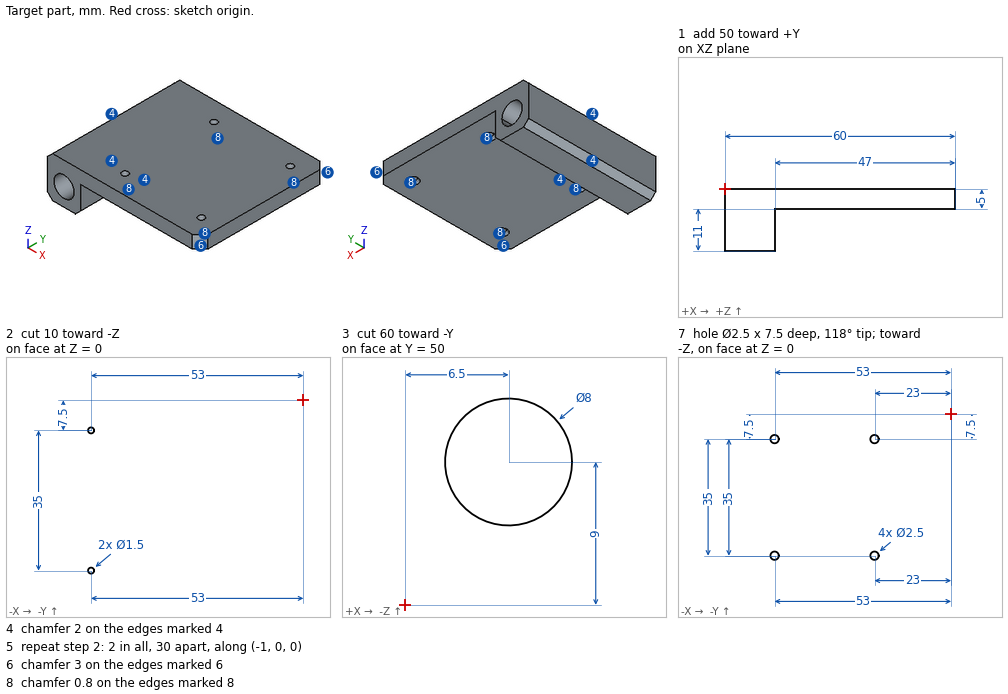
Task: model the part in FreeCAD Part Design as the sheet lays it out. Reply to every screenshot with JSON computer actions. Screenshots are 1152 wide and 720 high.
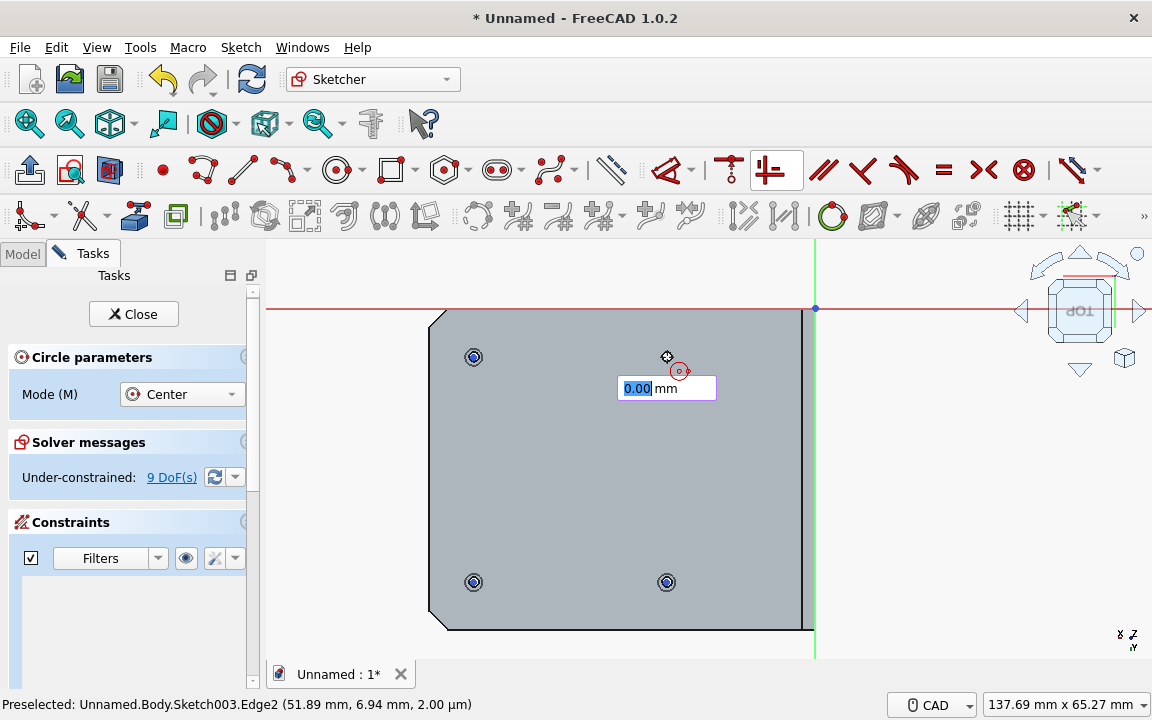
{"action": "scroll", "coordinate": [673, 351], "scroll_direction": "up", "scroll_amount": 4}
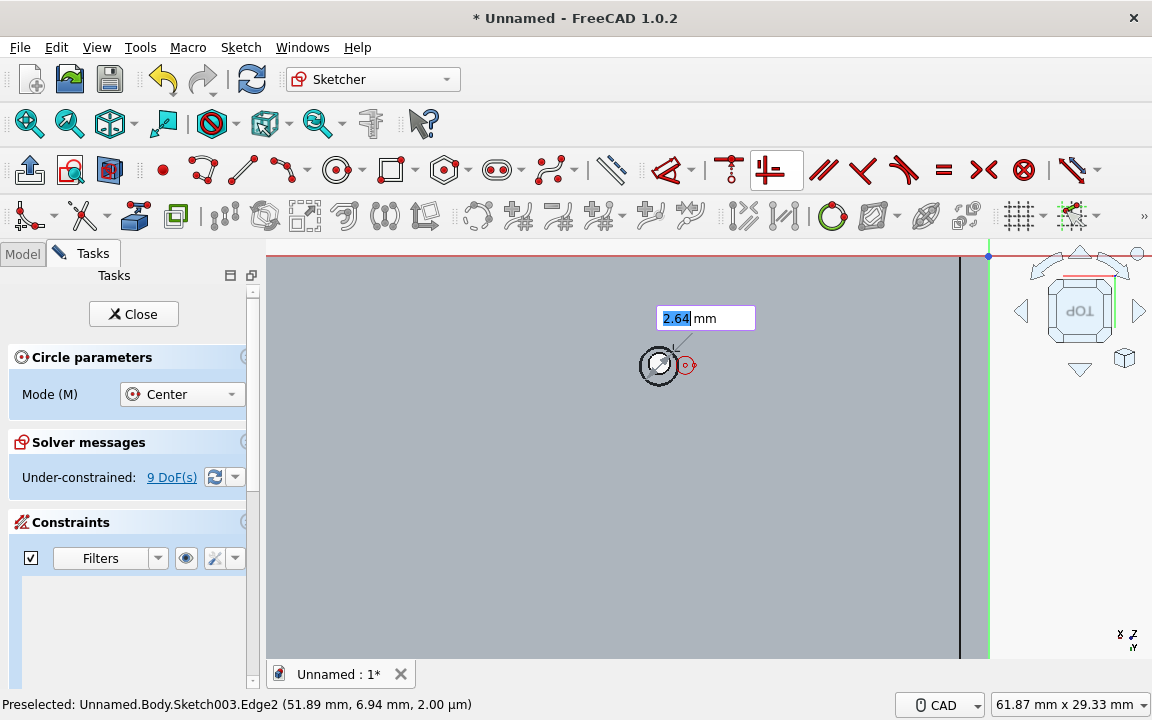
{"action": "left_click", "coordinate": [672, 351]}
{"action": "key", "text": "Escape"}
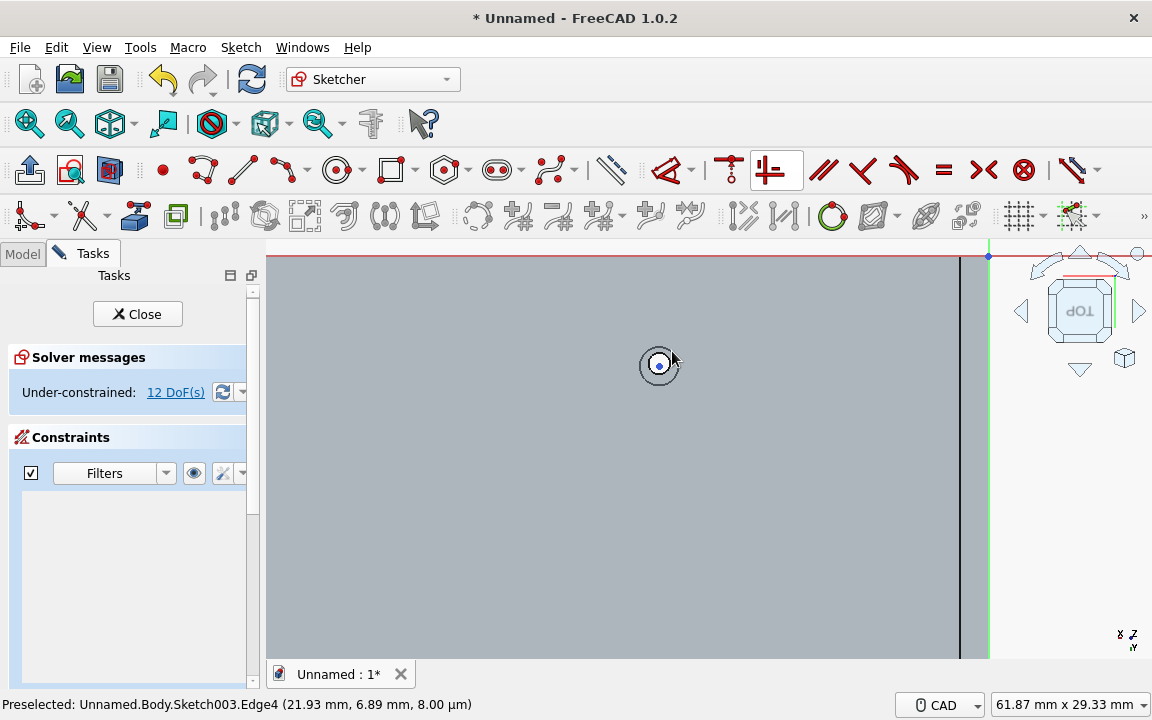
{"action": "scroll", "coordinate": [673, 351], "scroll_direction": "down", "scroll_amount": 4}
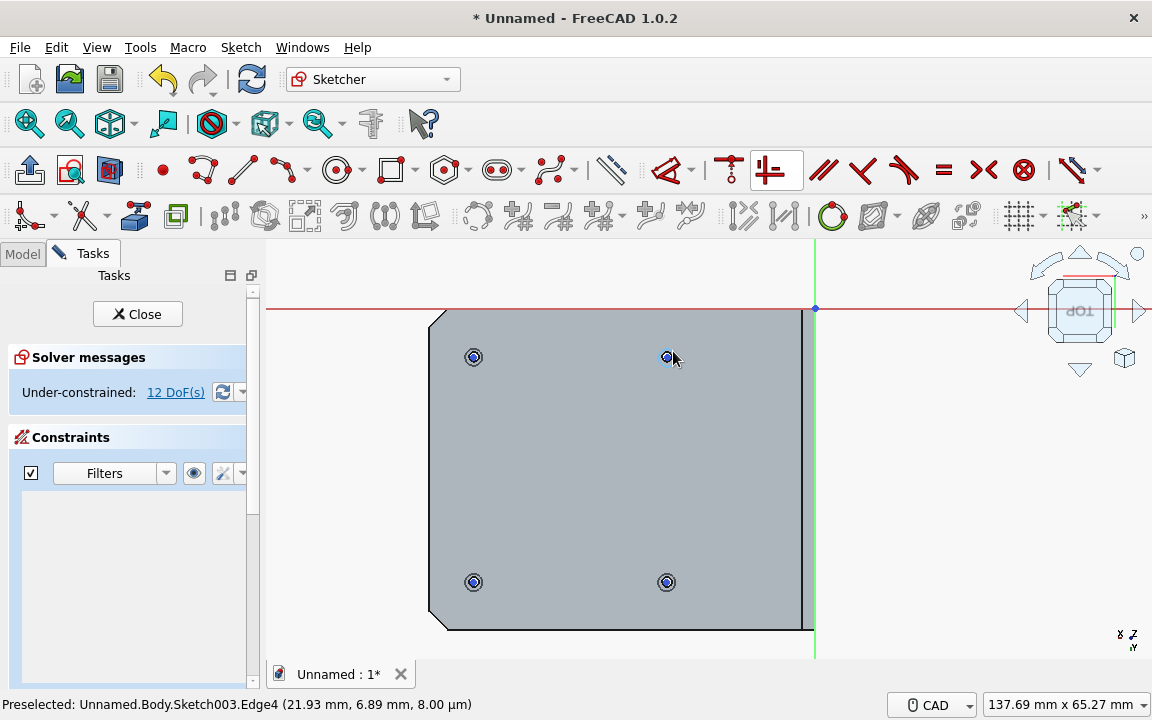
{"action": "scroll", "coordinate": [673, 576], "scroll_direction": "up", "scroll_amount": 3}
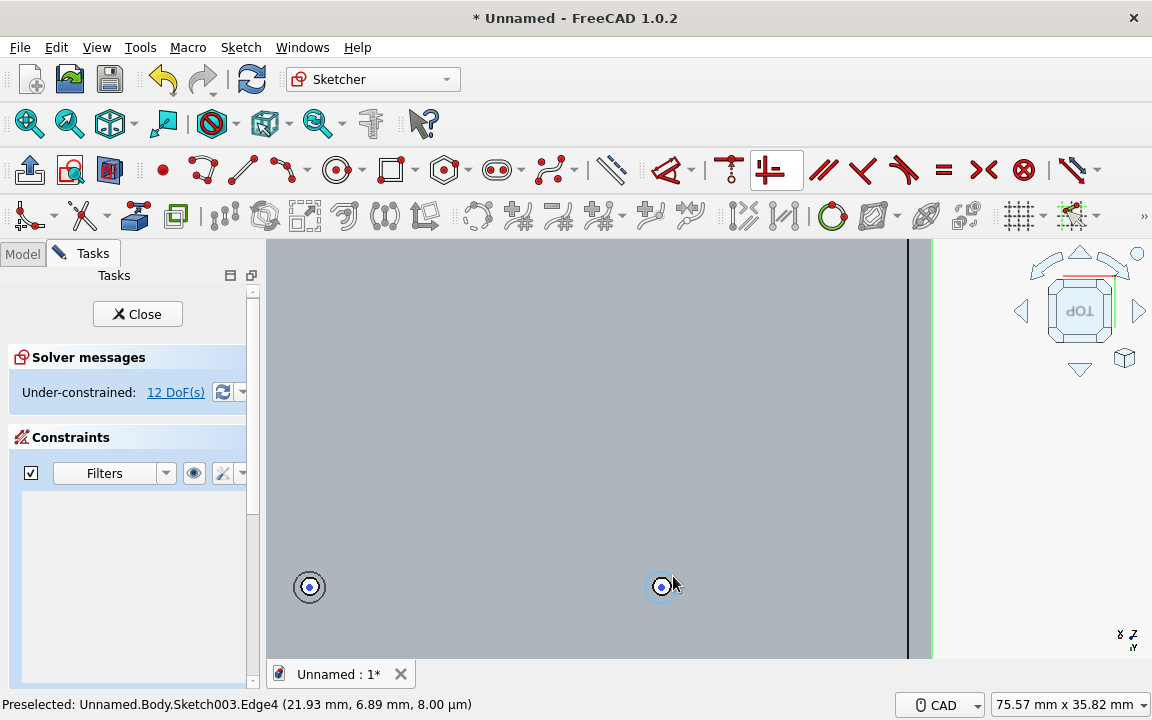
{"action": "left_click", "coordinate": [672, 576]}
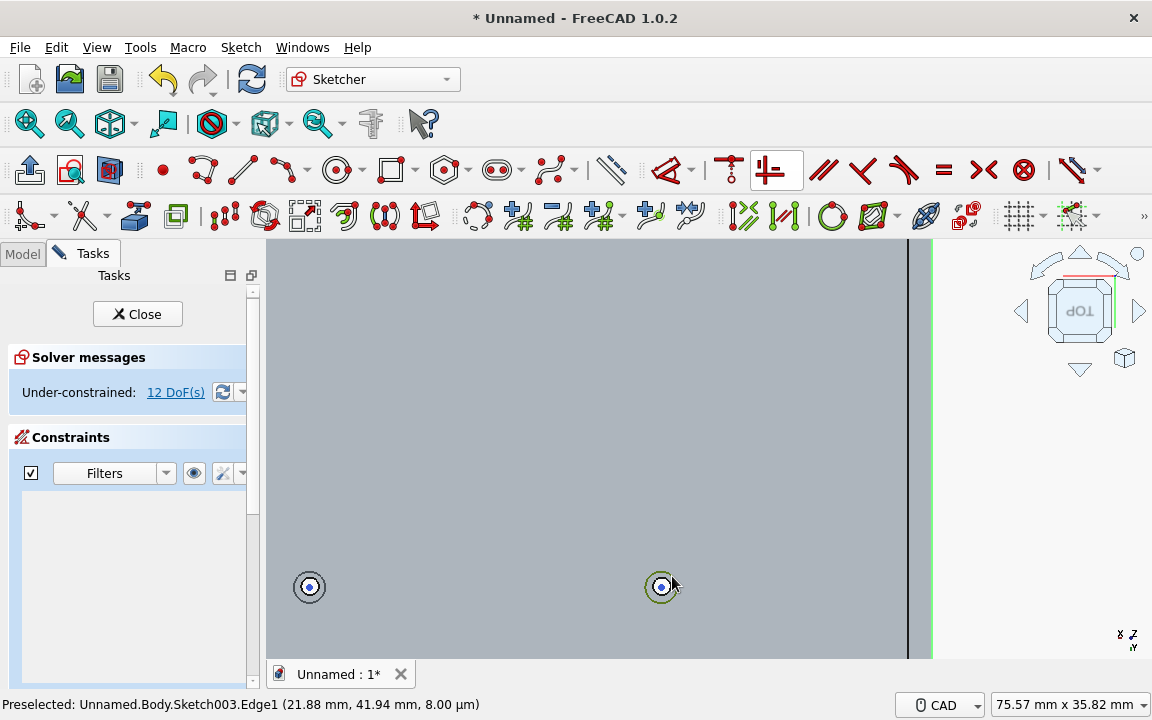
{"action": "left_click", "coordinate": [321, 576]}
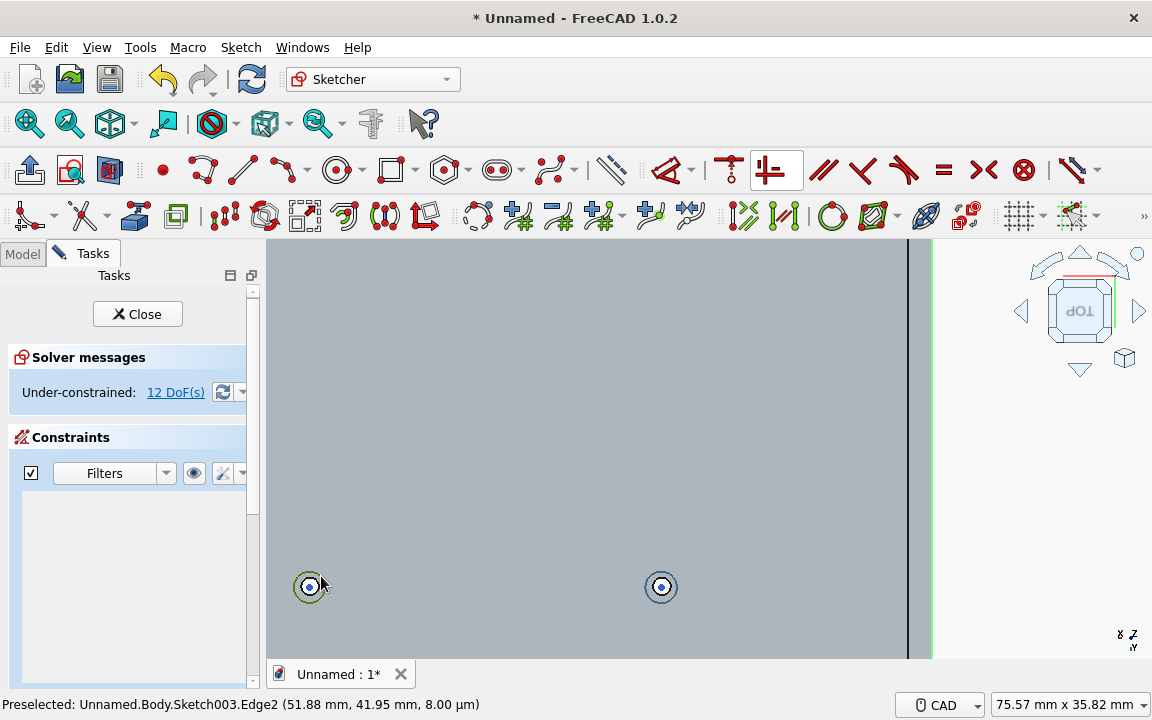
{"action": "scroll", "coordinate": [673, 576], "scroll_direction": "down", "scroll_amount": 3}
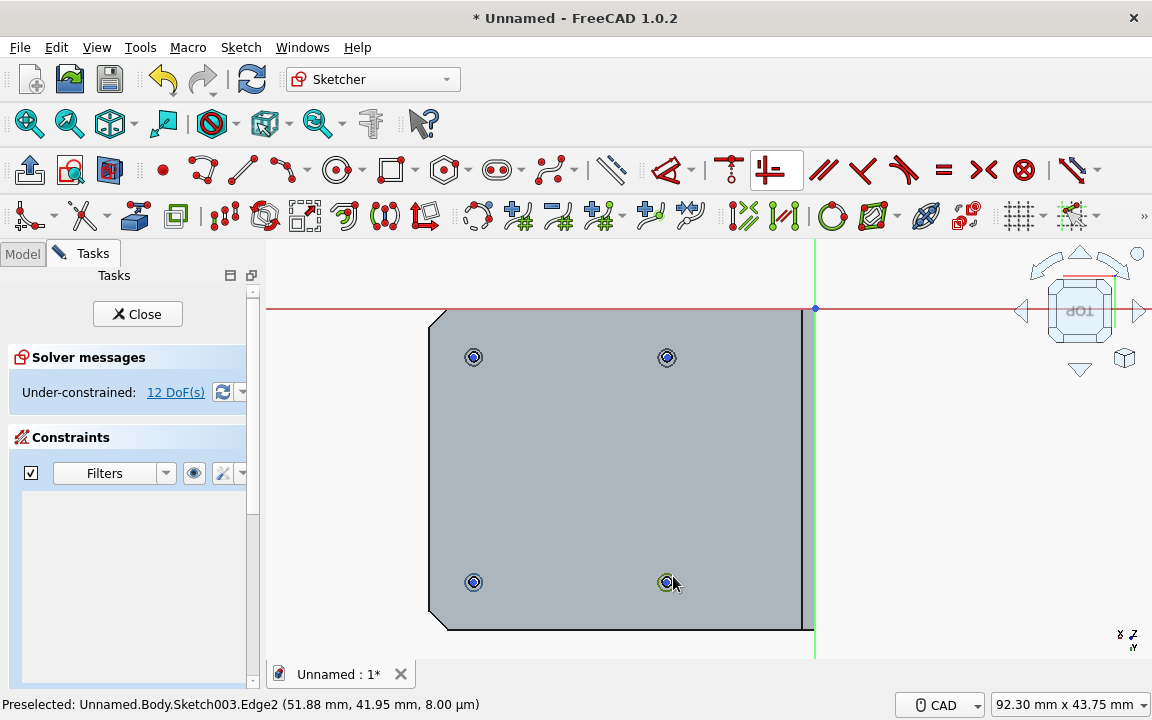
{"action": "scroll", "coordinate": [480, 351], "scroll_direction": "up", "scroll_amount": 3}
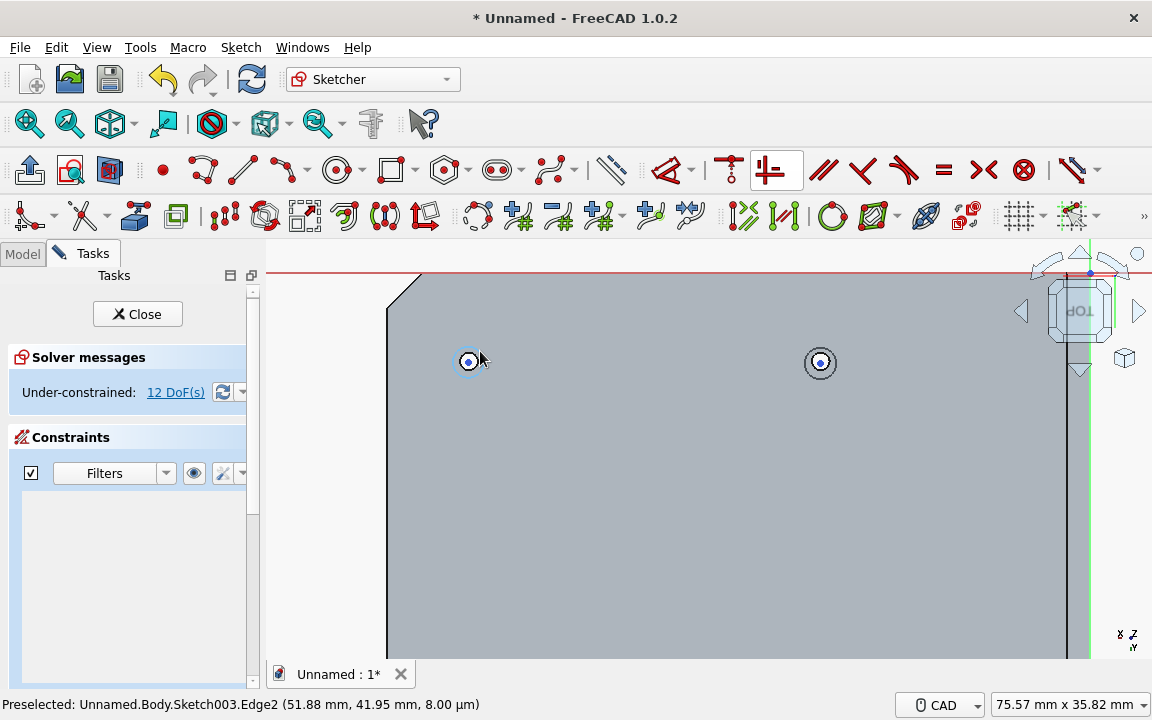
{"action": "left_click", "coordinate": [479, 351]}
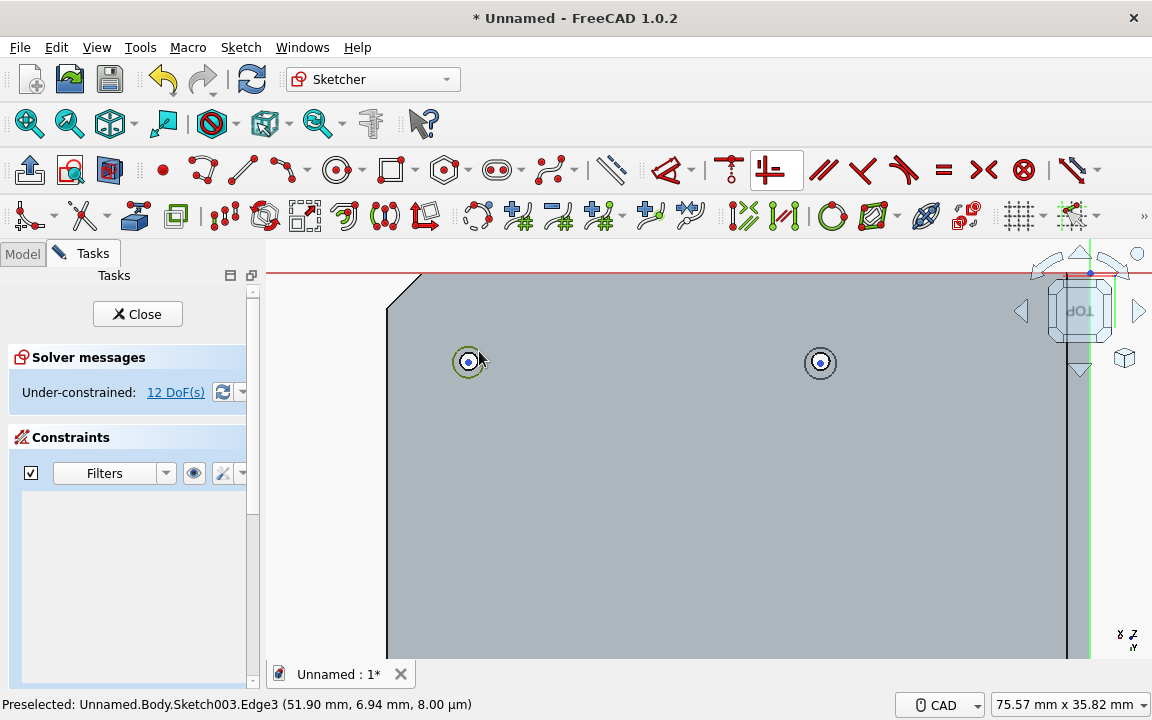
{"action": "left_click", "coordinate": [832, 352]}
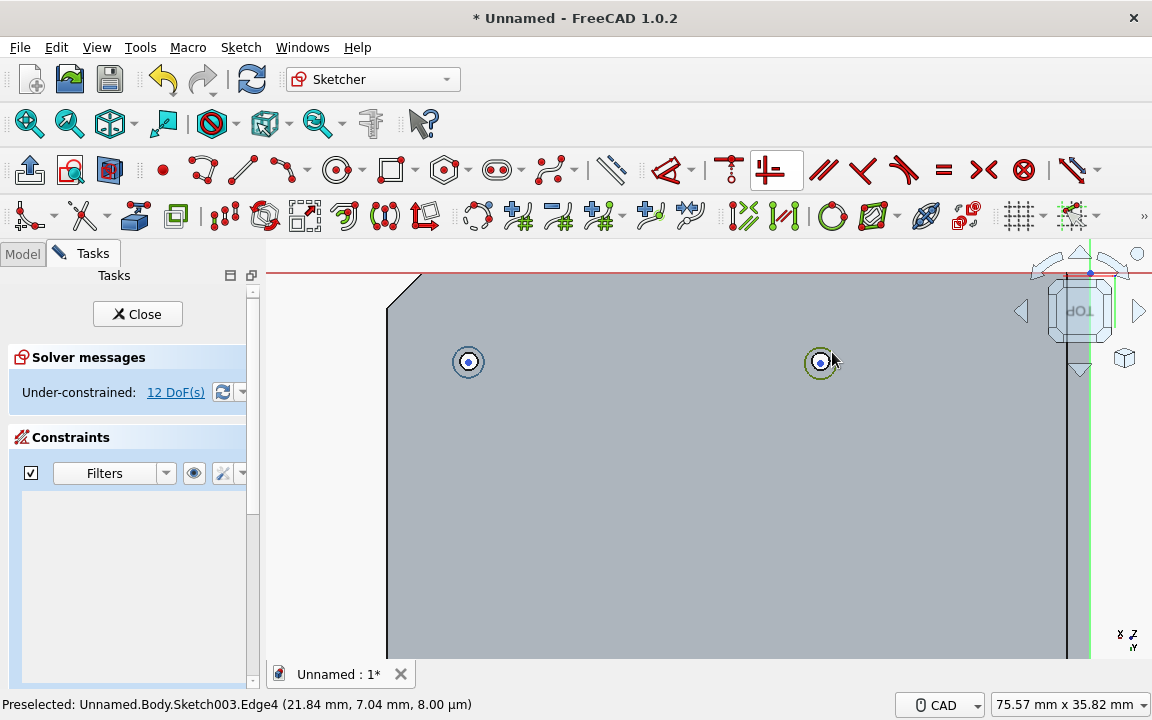
{"action": "key", "text": "e"}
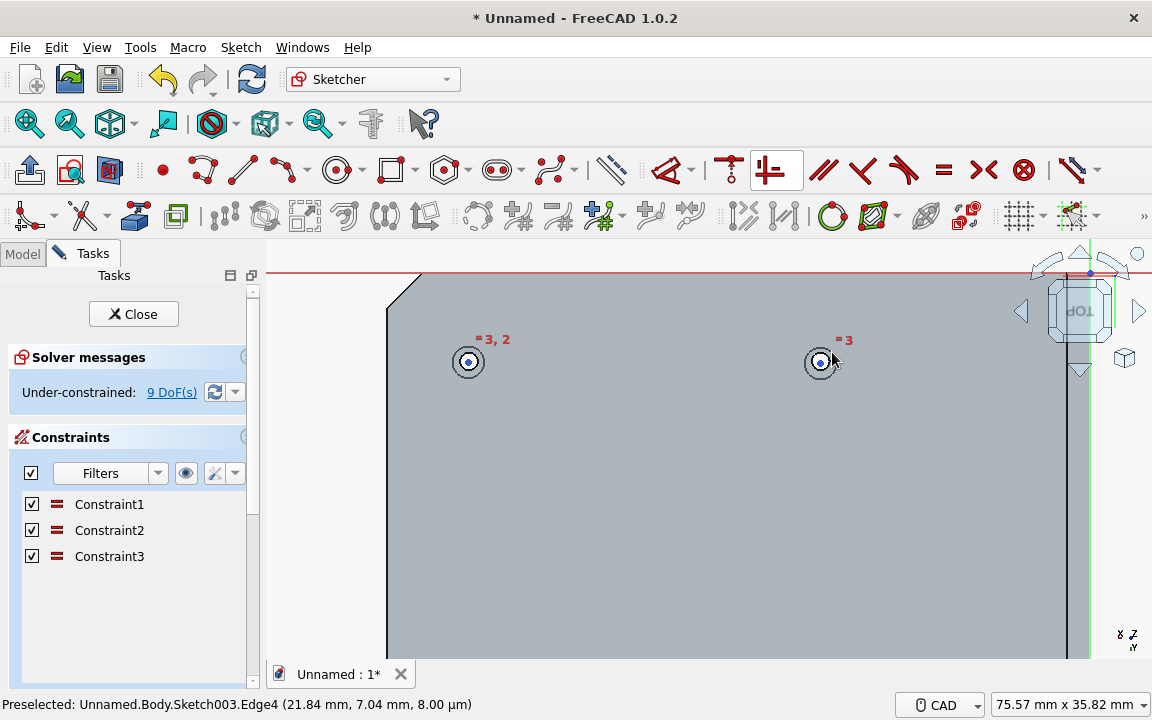
{"action": "left_click", "coordinate": [666, 170]}